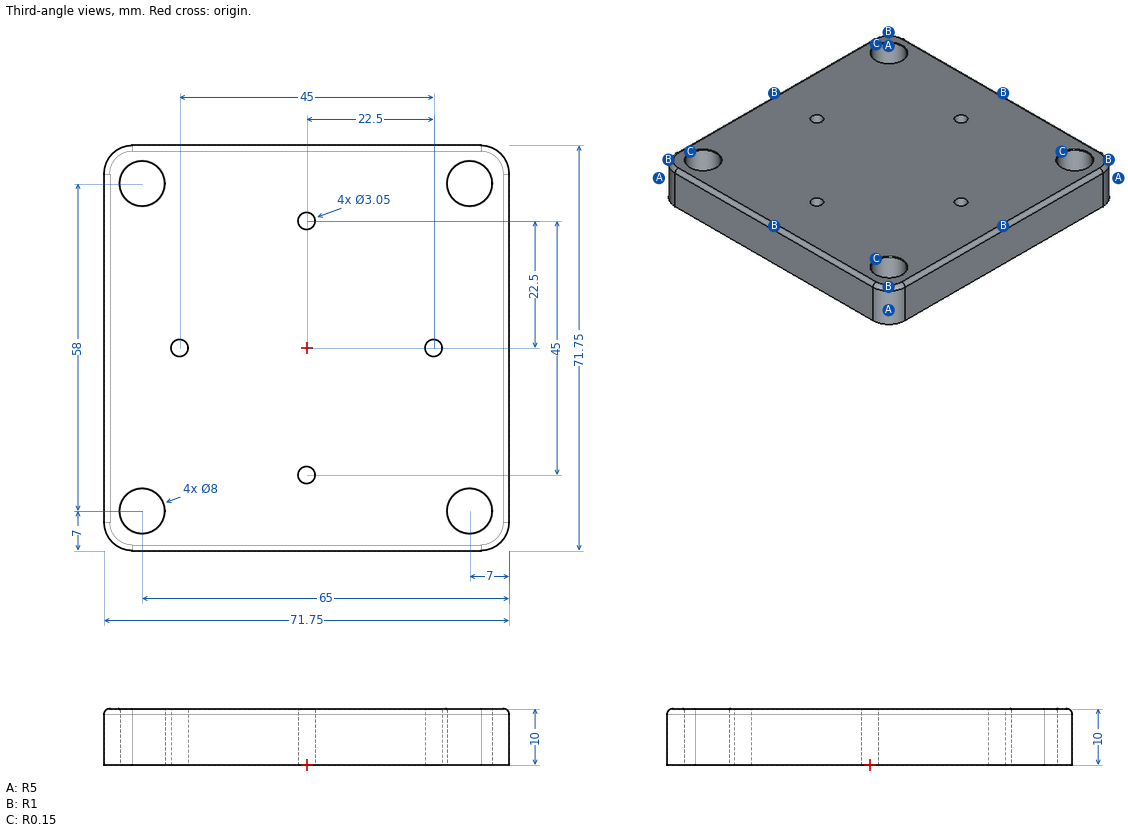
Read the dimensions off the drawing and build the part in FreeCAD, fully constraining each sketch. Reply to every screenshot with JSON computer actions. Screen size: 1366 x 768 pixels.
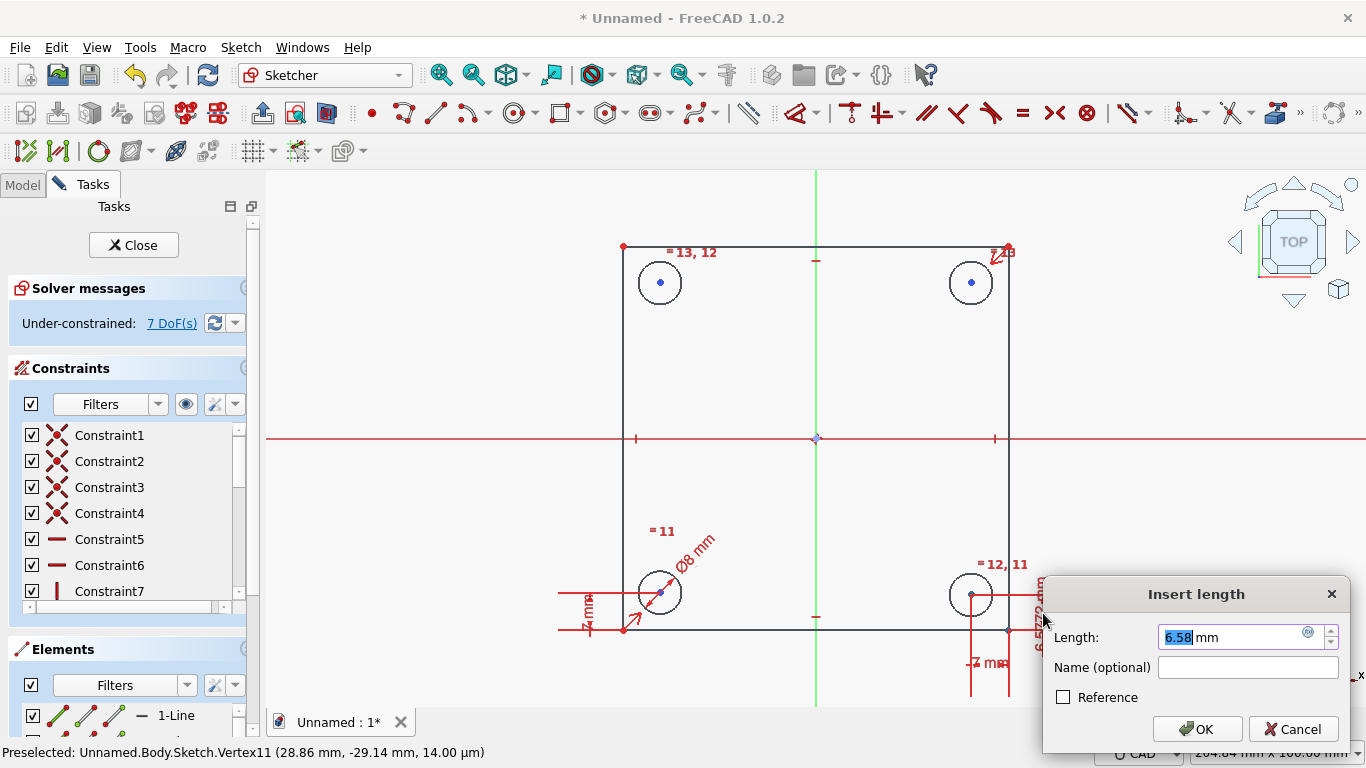
{"action": "type", "text": "7"}
{"action": "key", "text": "Return"}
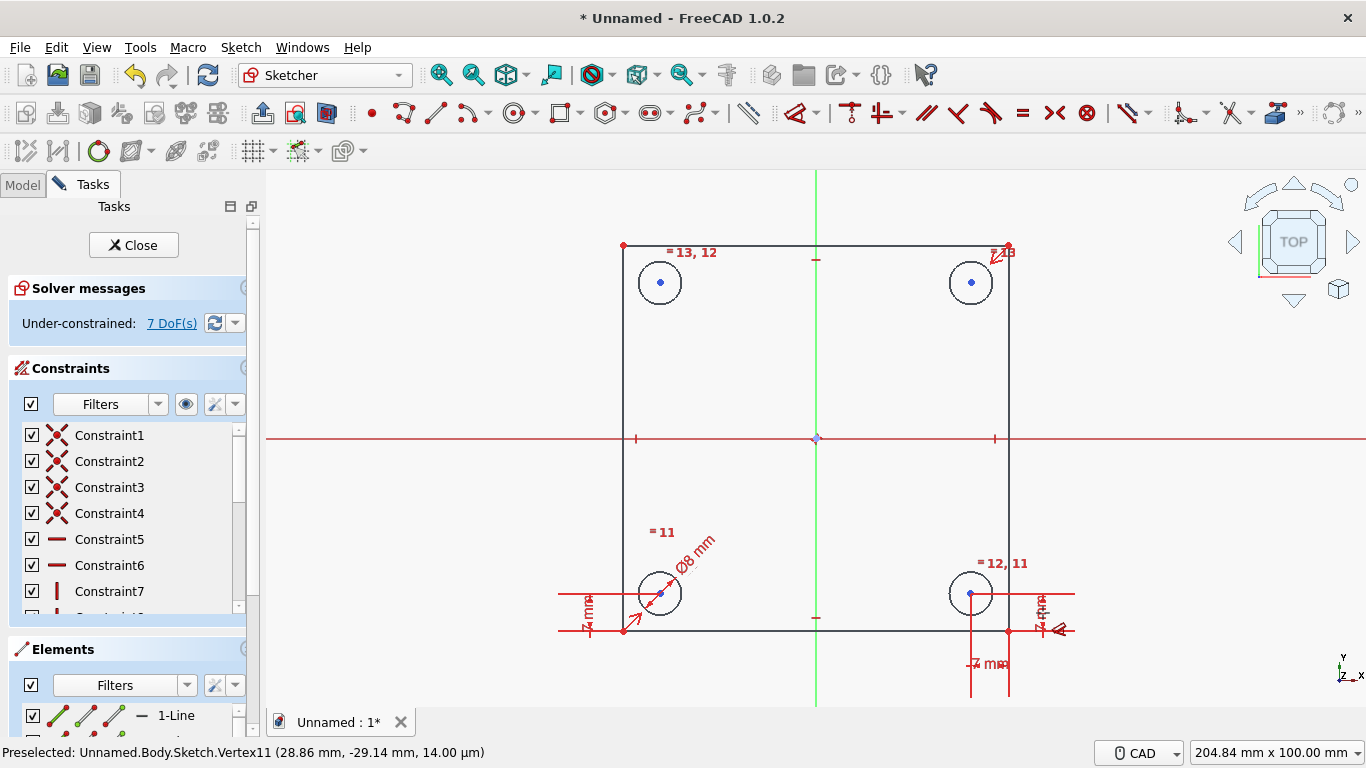
{"action": "left_click", "coordinate": [1009, 246]}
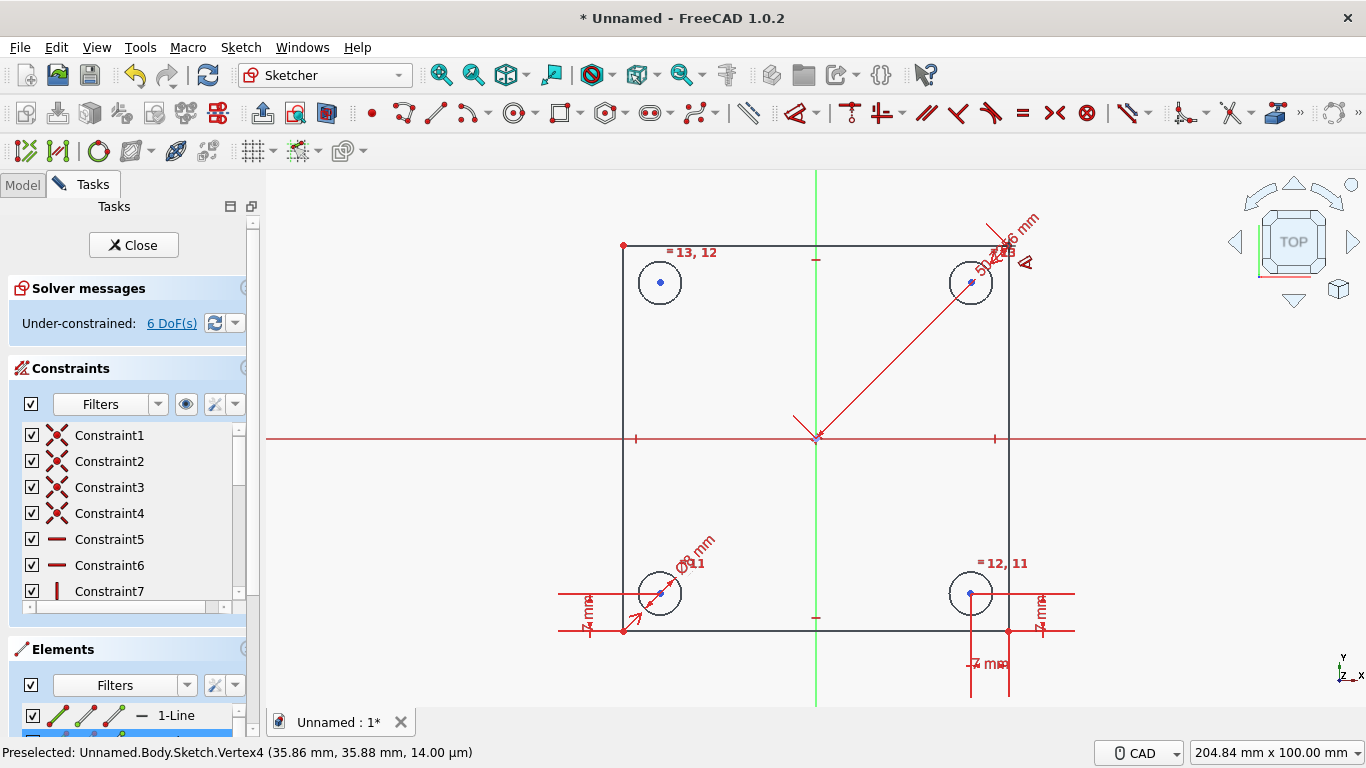
{"action": "left_click", "coordinate": [971, 283]}
{"action": "left_click", "coordinate": [990, 212]}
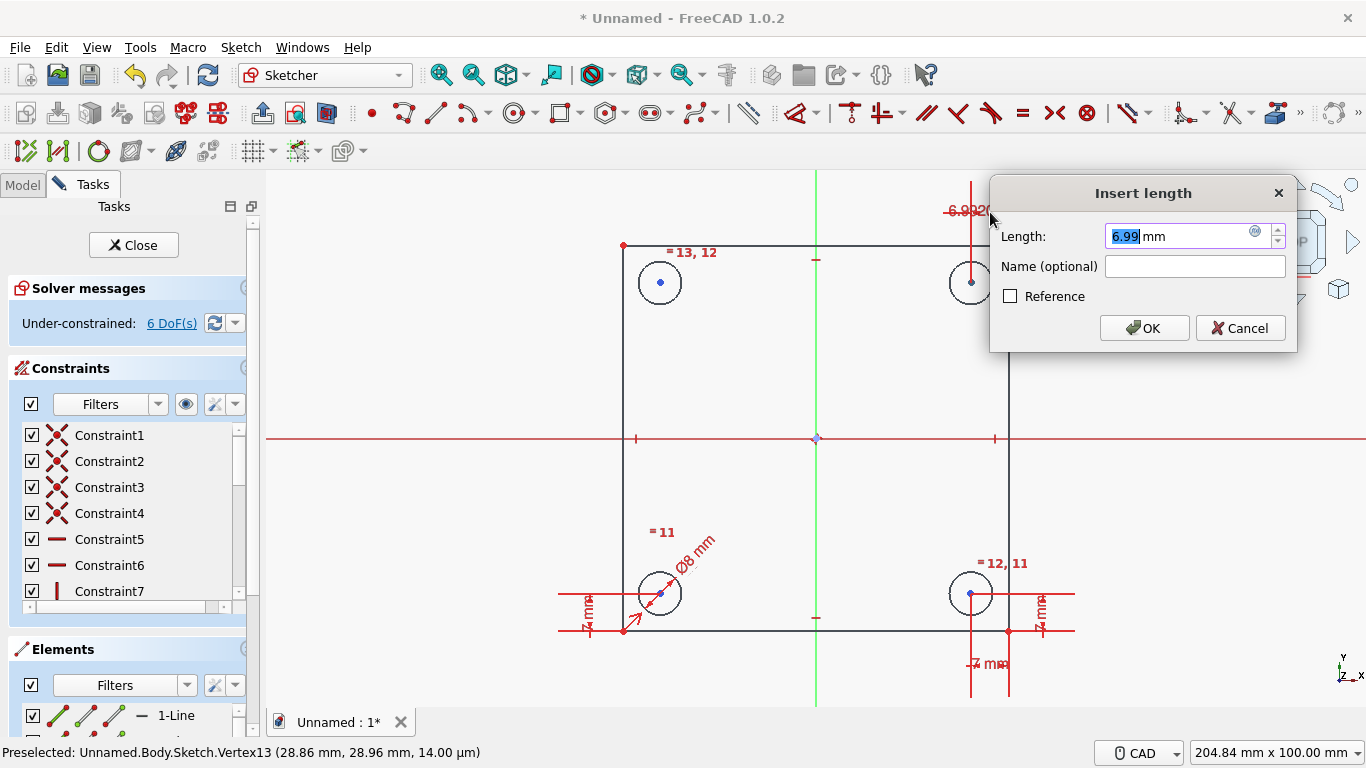
{"action": "type", "text": "7"}
{"action": "key", "text": "Return"}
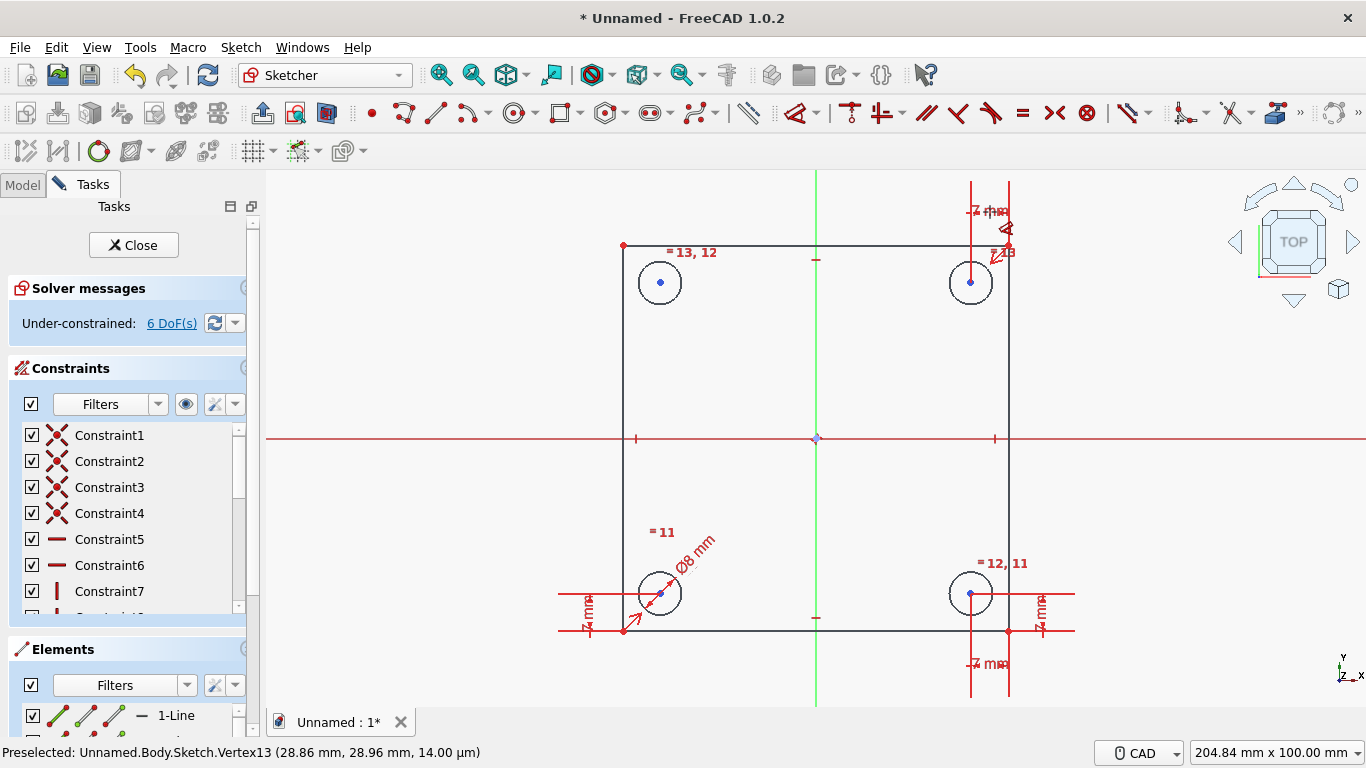
{"action": "left_click", "coordinate": [1009, 631]}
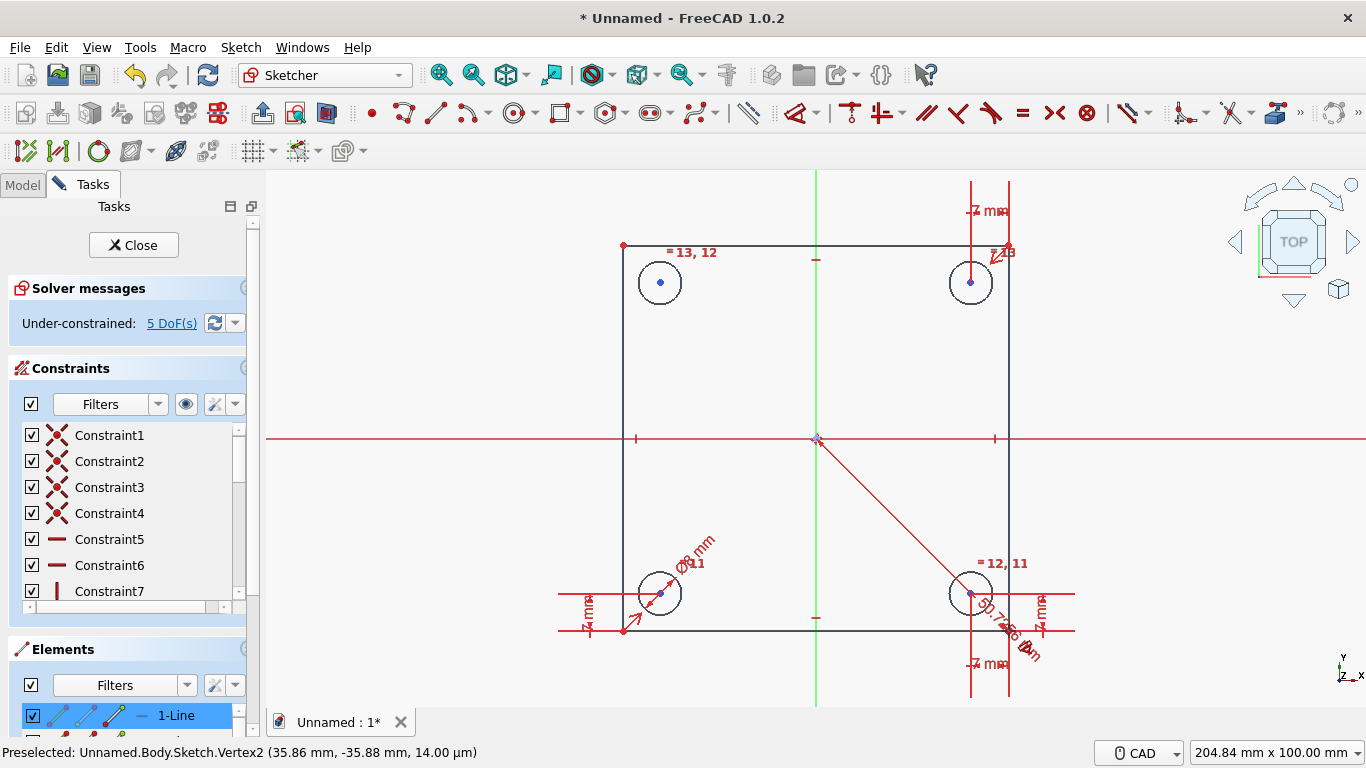
{"action": "left_click", "coordinate": [660, 594]}
{"action": "left_click", "coordinate": [834, 665]}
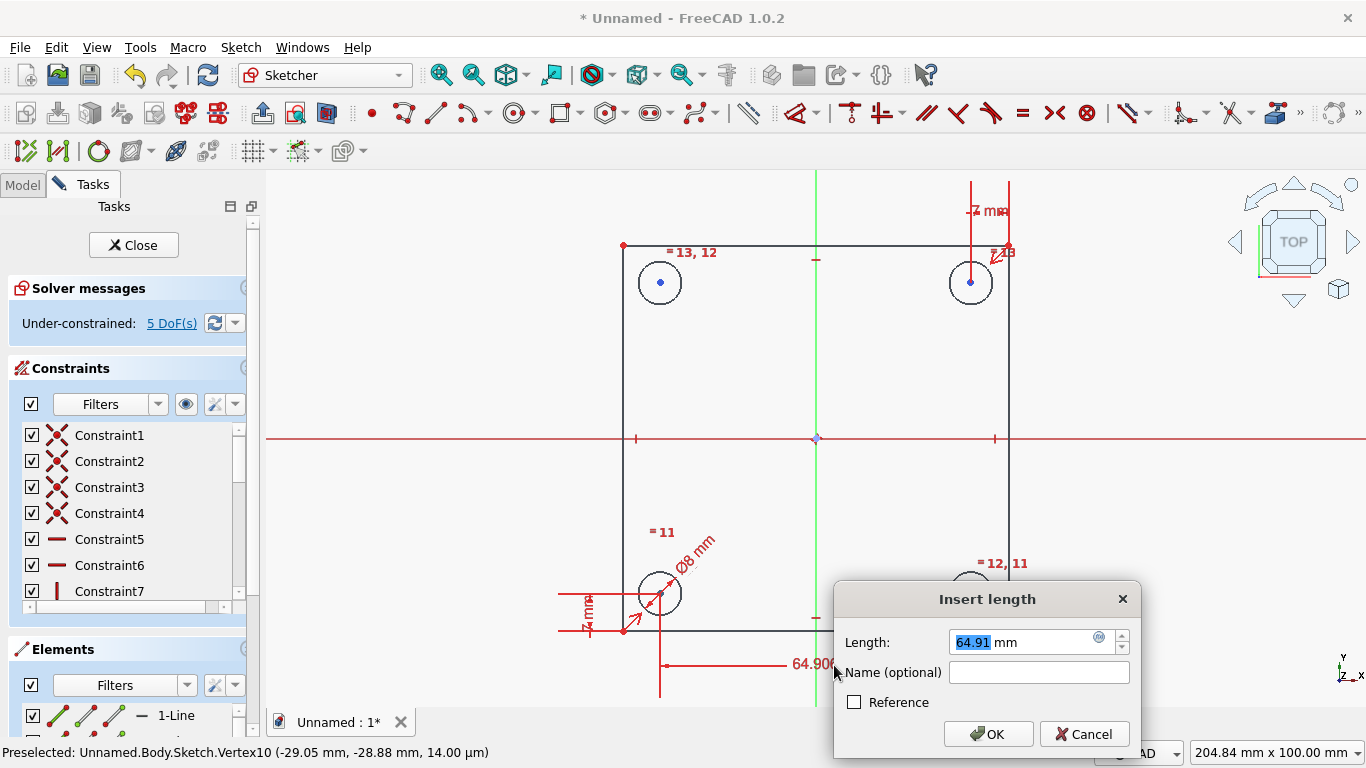
{"action": "type", "text": "65"}
{"action": "key", "text": "Return"}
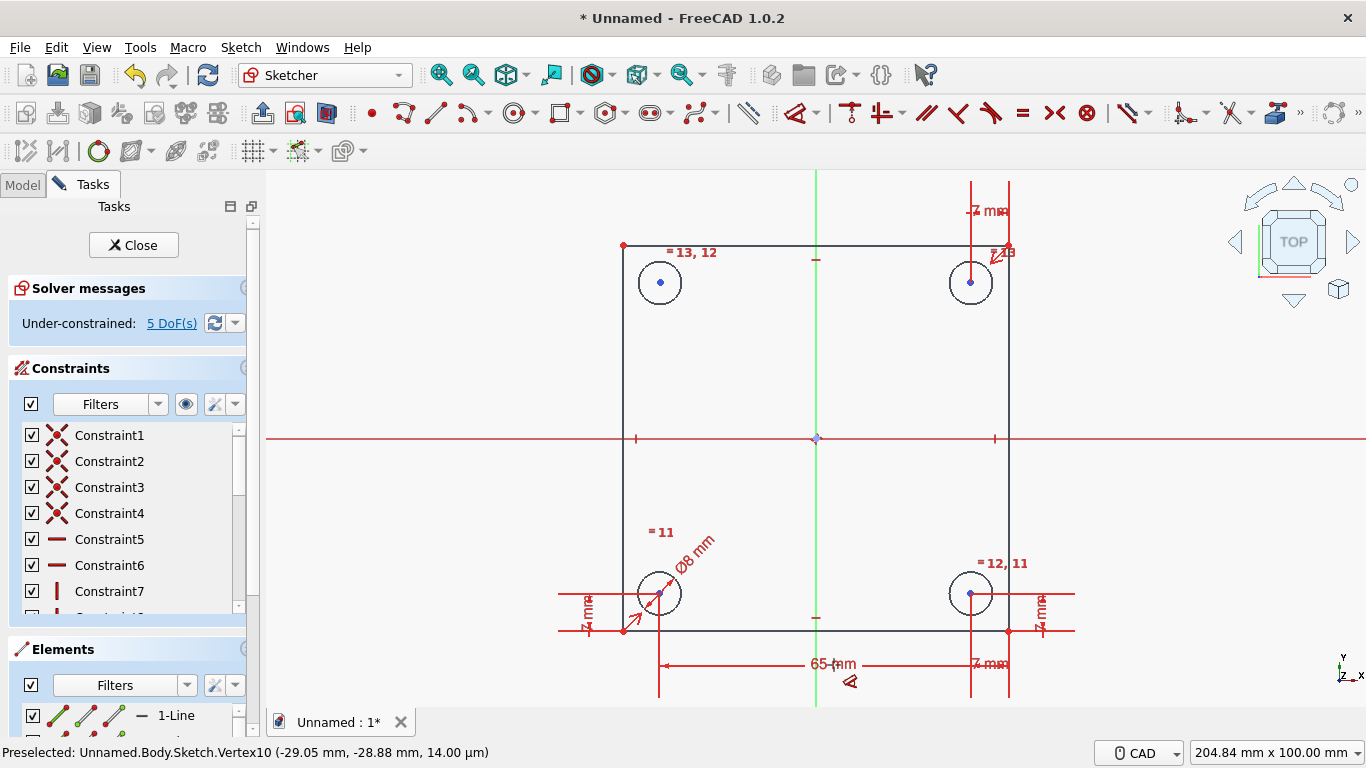
{"action": "left_click", "coordinate": [1009, 246]}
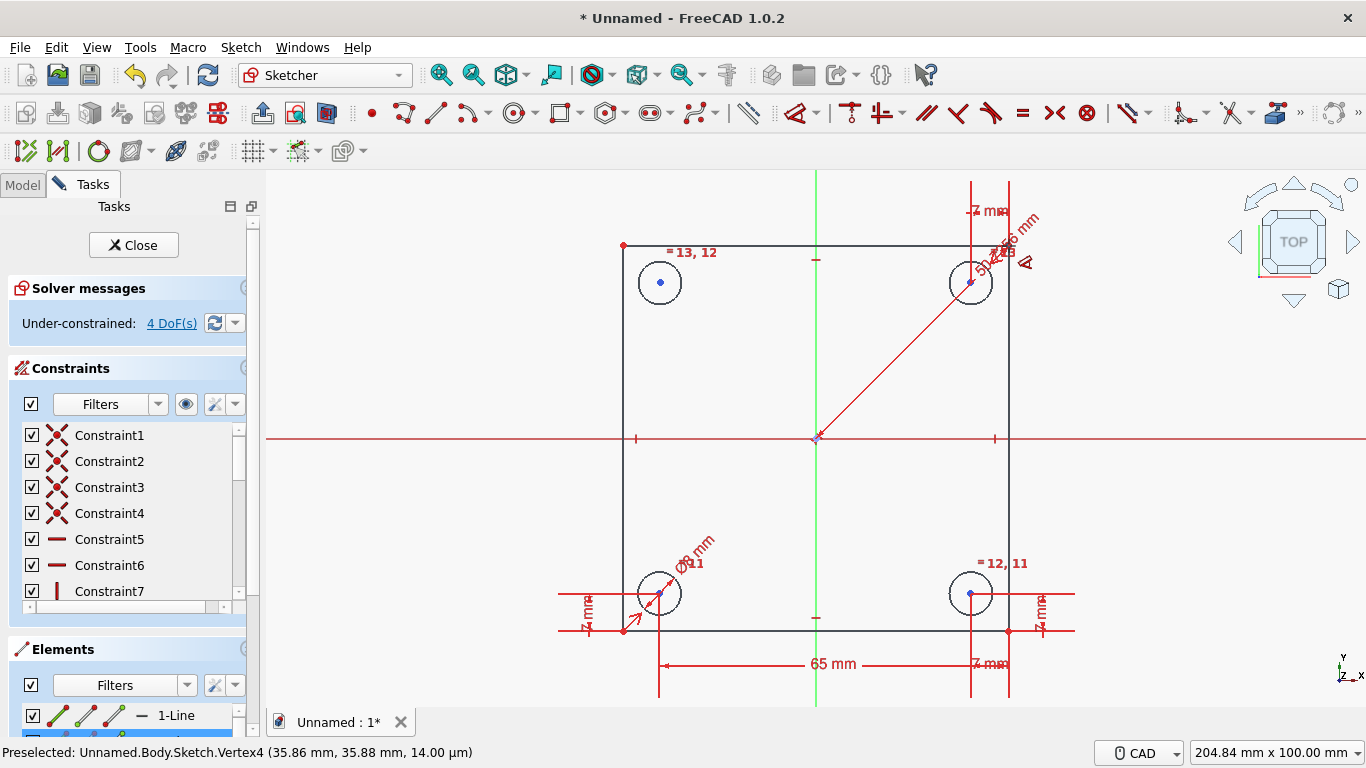
{"action": "left_click", "coordinate": [660, 283]}
{"action": "left_click", "coordinate": [834, 212]}